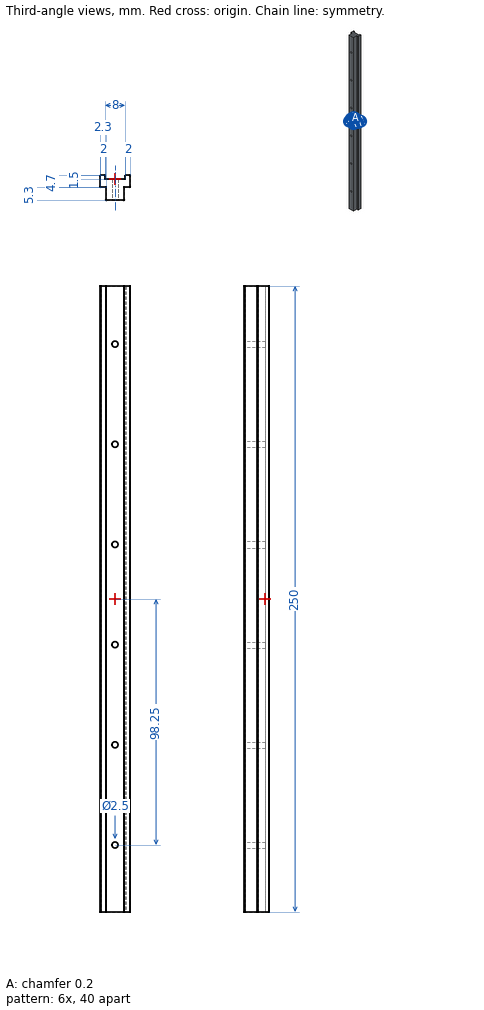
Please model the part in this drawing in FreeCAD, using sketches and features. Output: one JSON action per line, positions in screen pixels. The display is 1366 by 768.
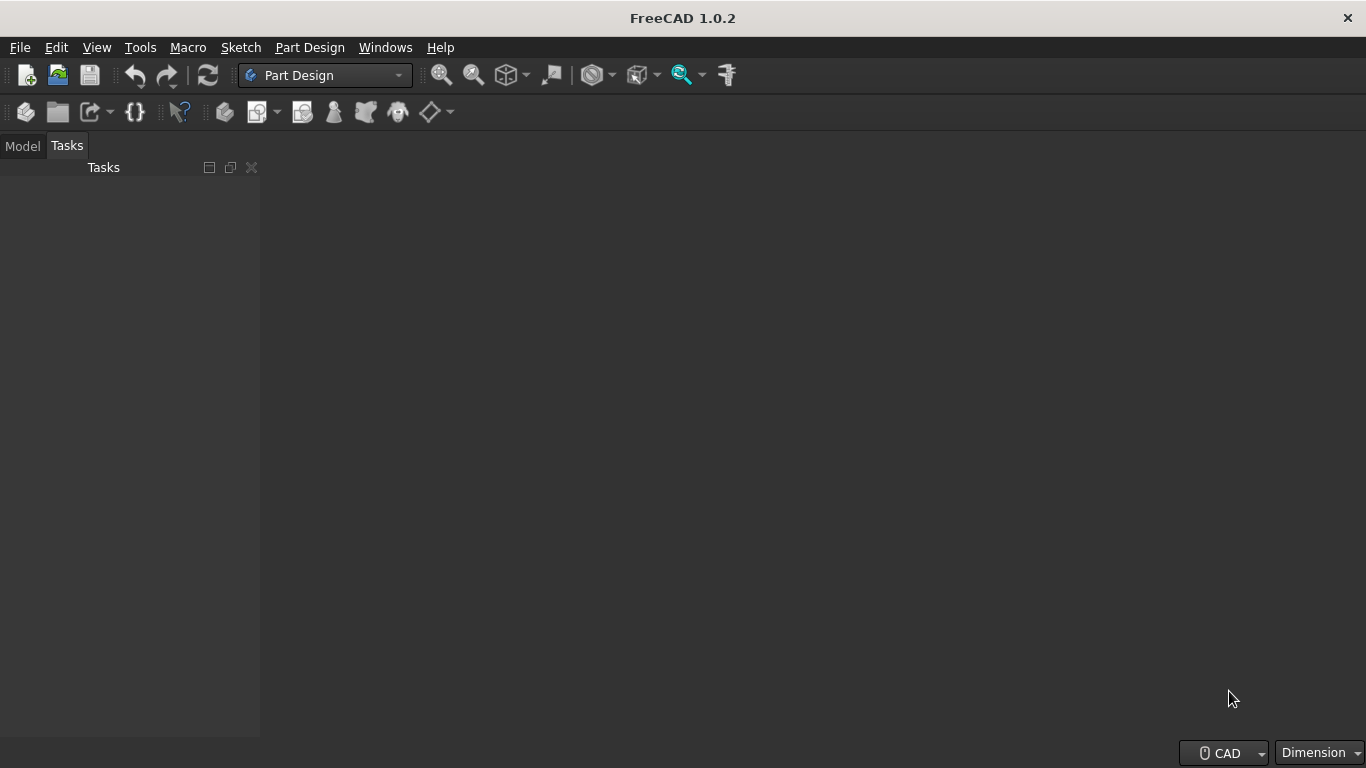
{"action": "left_click", "coordinate": [1098, 76]}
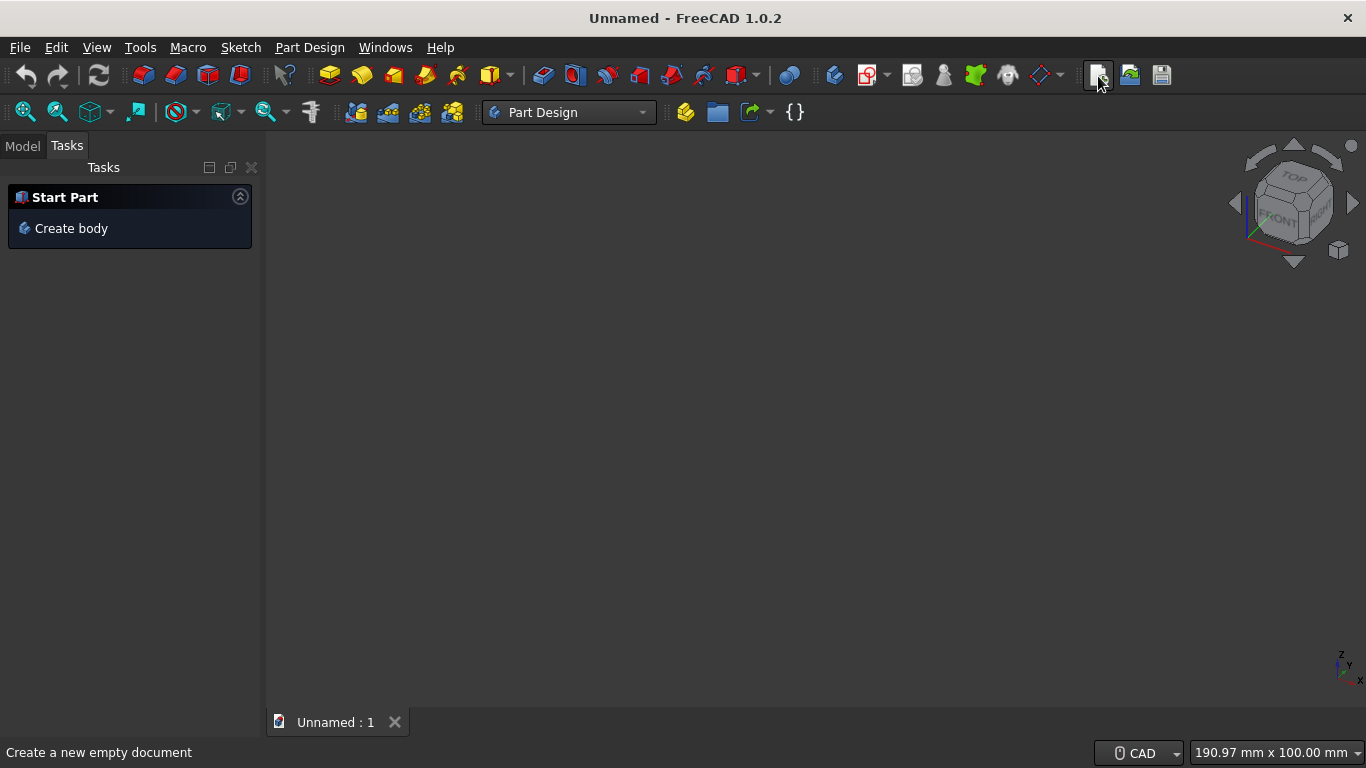
{"action": "left_click", "coordinate": [868, 76]}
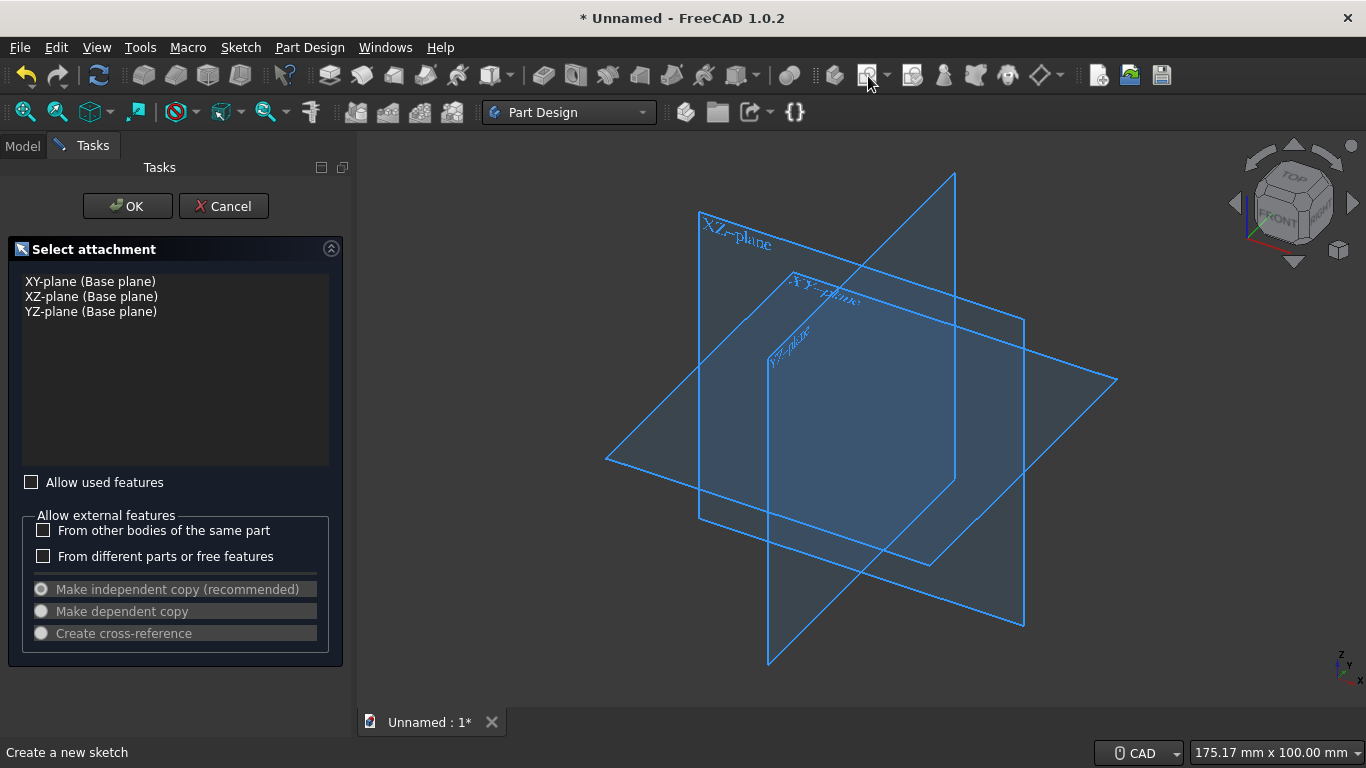
{"action": "left_click", "coordinate": [82, 282]}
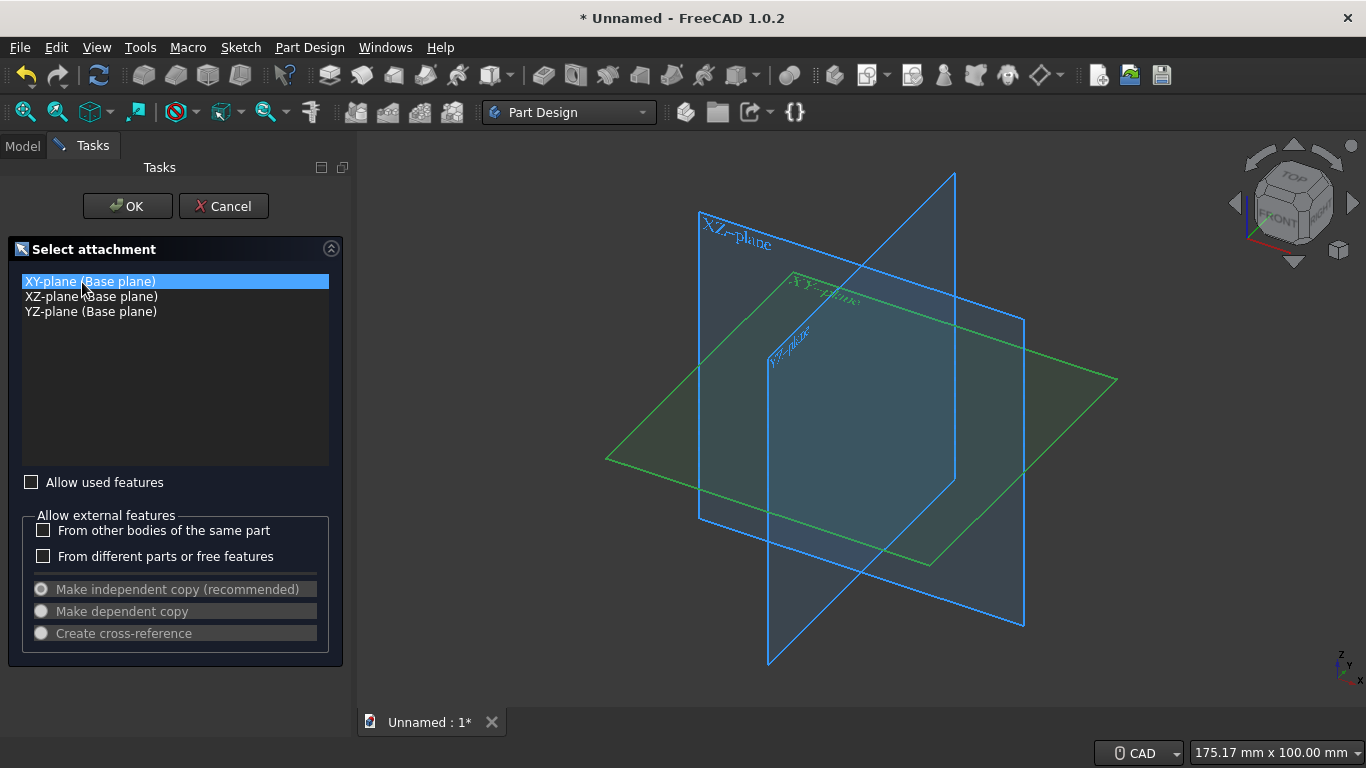
{"action": "left_click", "coordinate": [128, 206]}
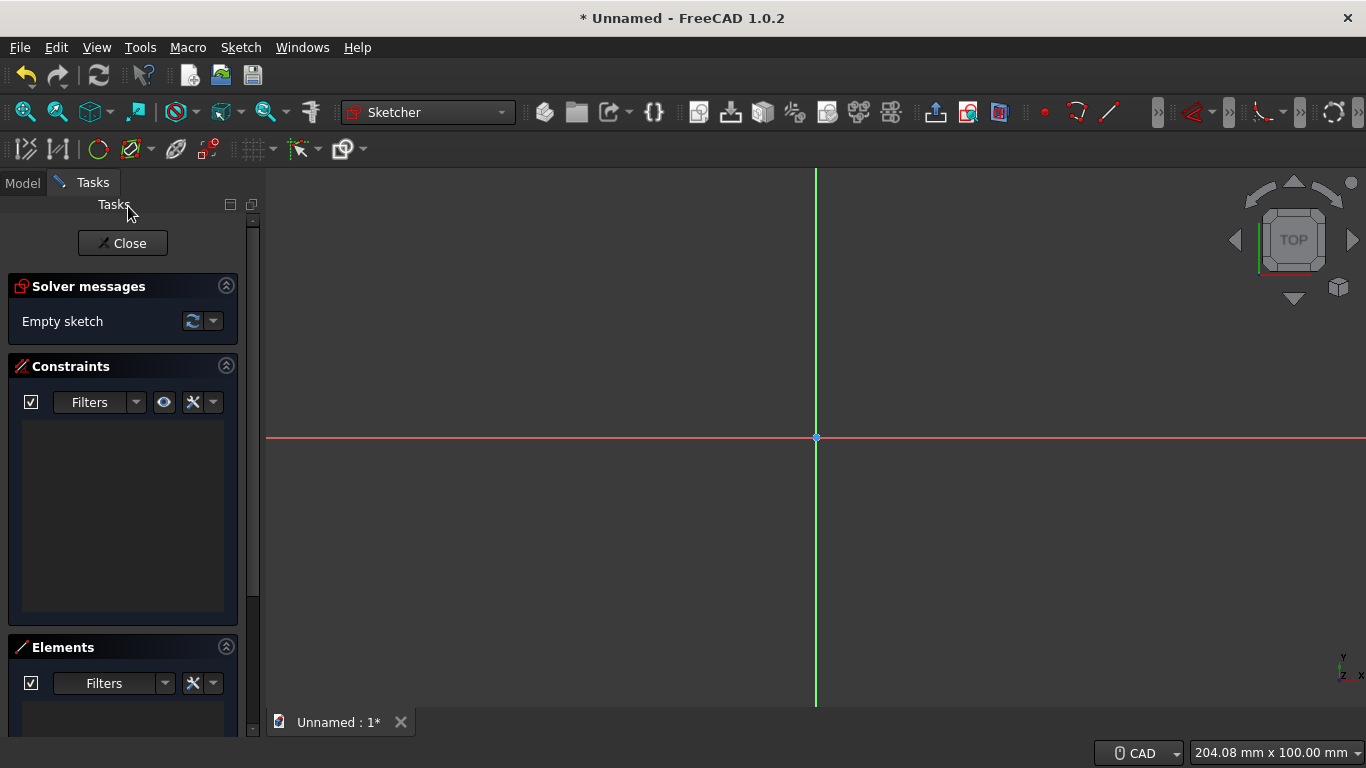
{"action": "scroll", "coordinate": [830, 460], "scroll_direction": "up", "scroll_amount": 9}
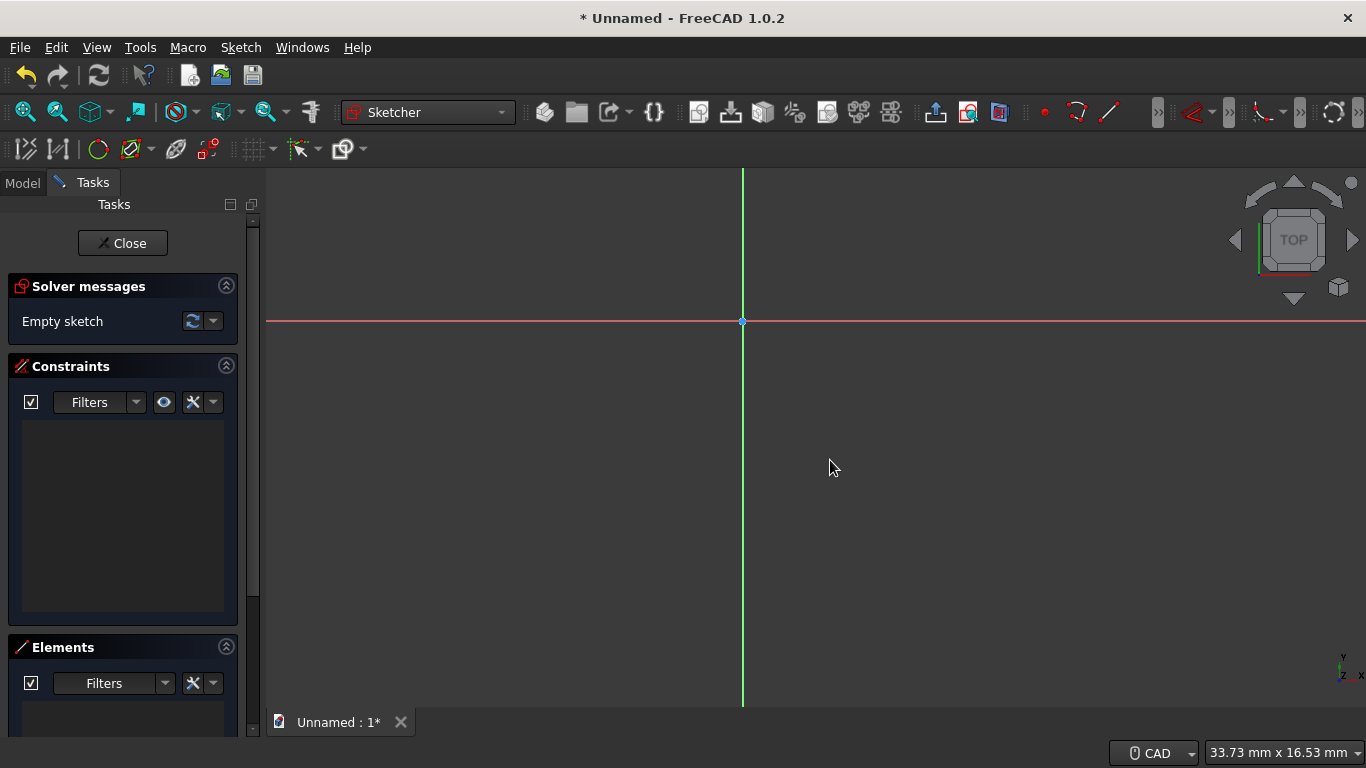
{"action": "left_click", "coordinate": [1078, 112]}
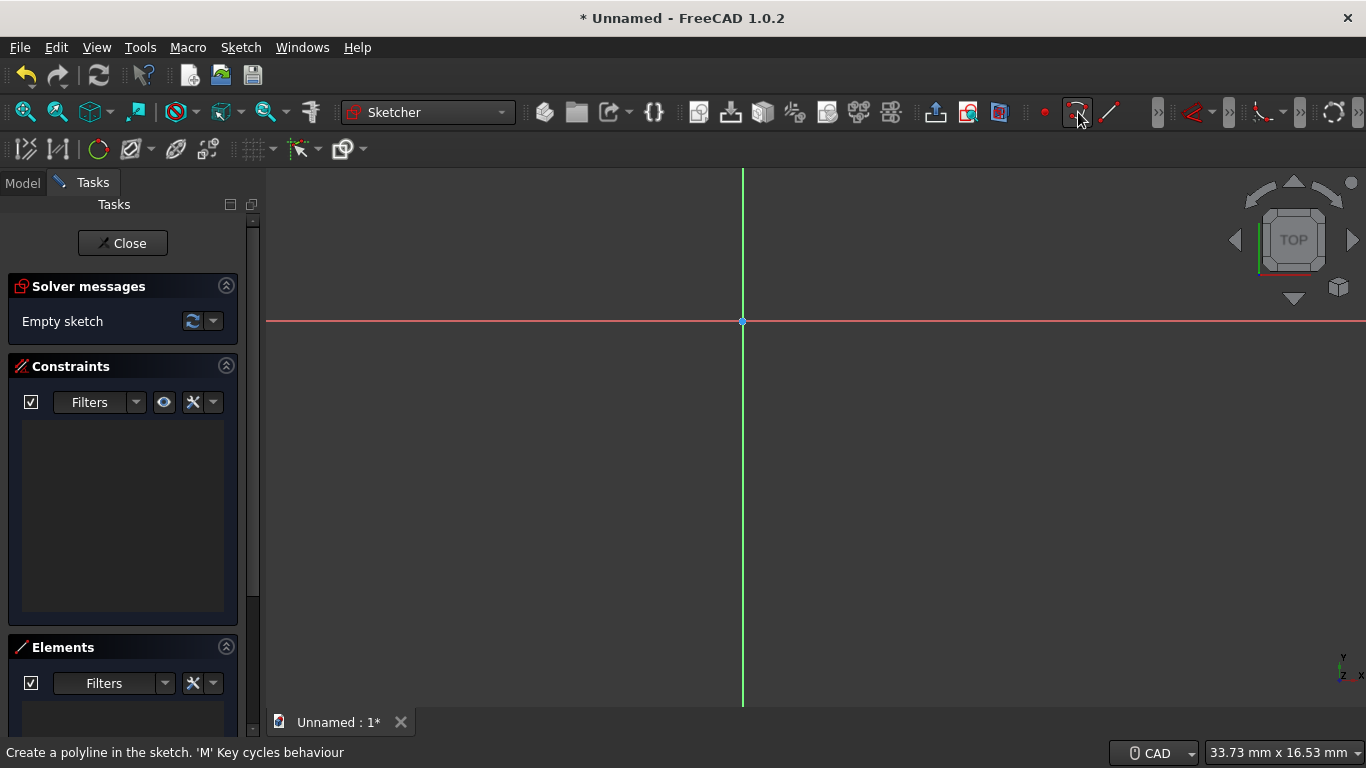
{"action": "left_click", "coordinate": [873, 321]}
{"action": "left_click", "coordinate": [612, 330]}
{"action": "left_click", "coordinate": [612, 272]}
{"action": "left_click", "coordinate": [547, 272]}
{"action": "left_click", "coordinate": [547, 425]}
{"action": "left_click", "coordinate": [622, 425]}
{"action": "left_click", "coordinate": [622, 598]}
{"action": "left_click", "coordinate": [863, 598]}
{"action": "left_click", "coordinate": [863, 425]}
{"action": "left_click", "coordinate": [938, 425]}
{"action": "left_click", "coordinate": [938, 272]}
{"action": "left_click", "coordinate": [873, 272]}
{"action": "left_click", "coordinate": [873, 321]}
{"action": "key", "text": "Escape"}
{"action": "key", "text": "Escape"}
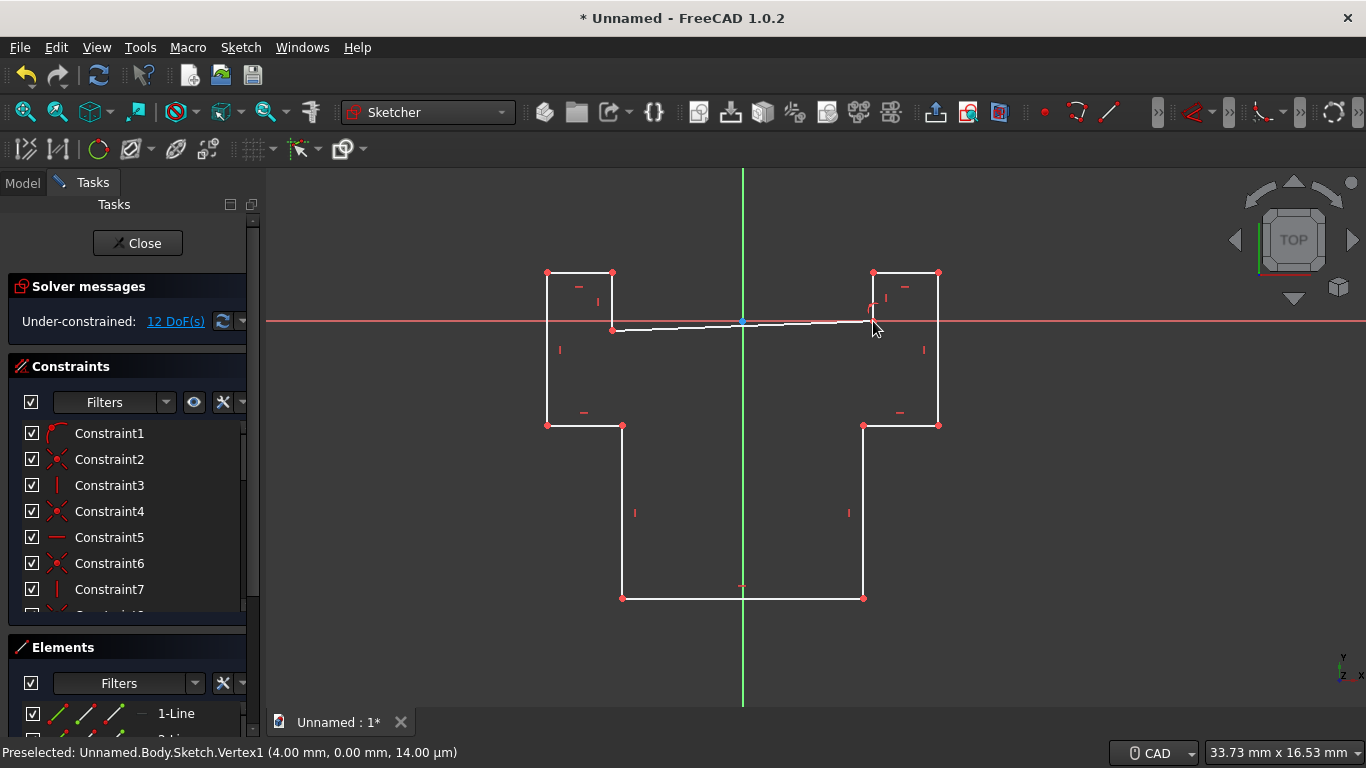
{"action": "left_click", "coordinate": [795, 324]}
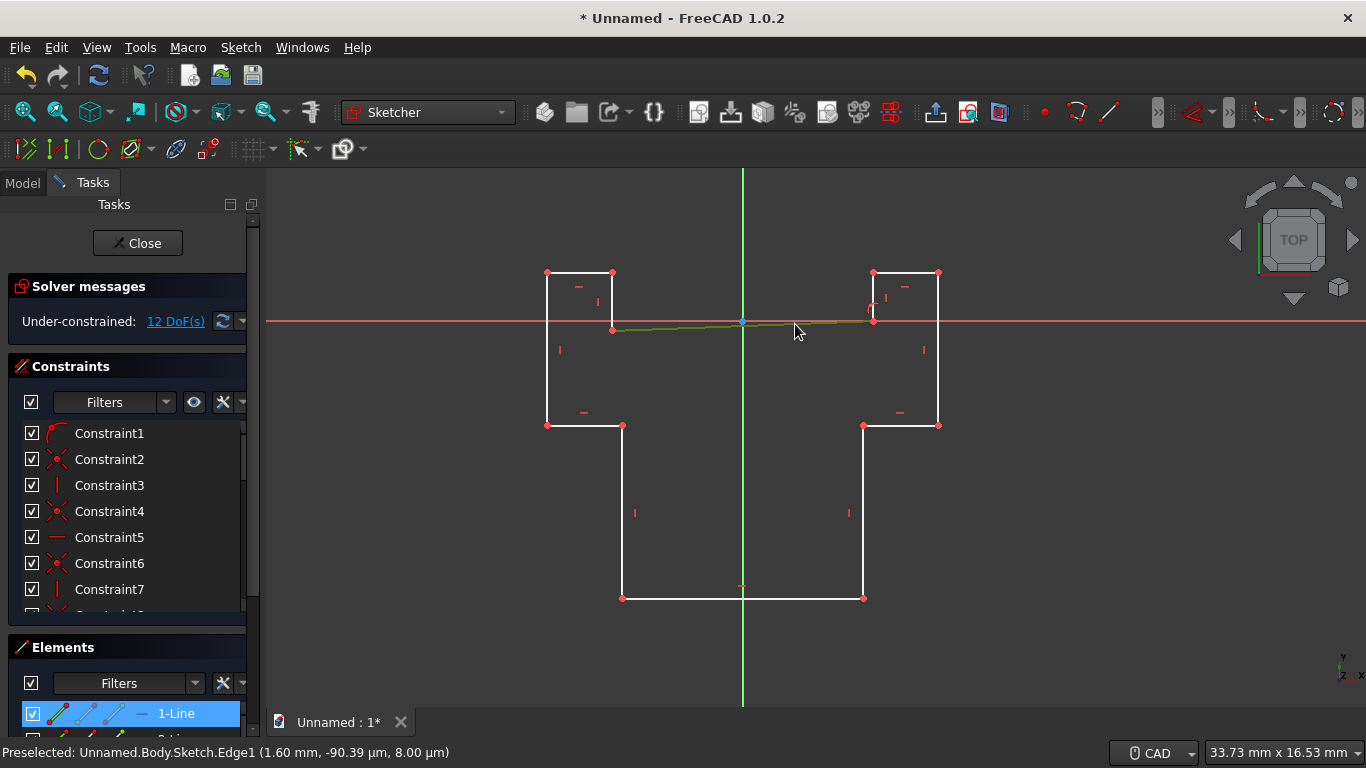
{"action": "key", "text": "h"}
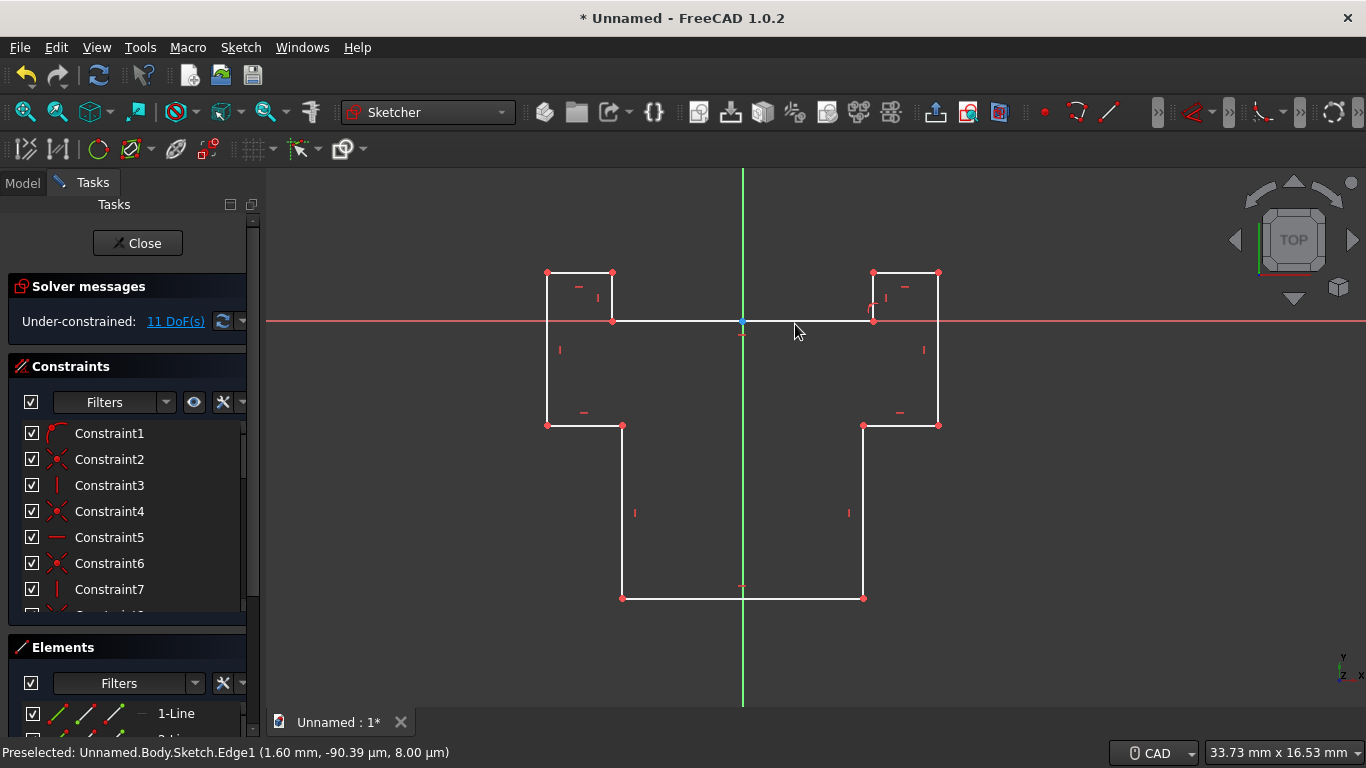
{"action": "left_click", "coordinate": [622, 426]}